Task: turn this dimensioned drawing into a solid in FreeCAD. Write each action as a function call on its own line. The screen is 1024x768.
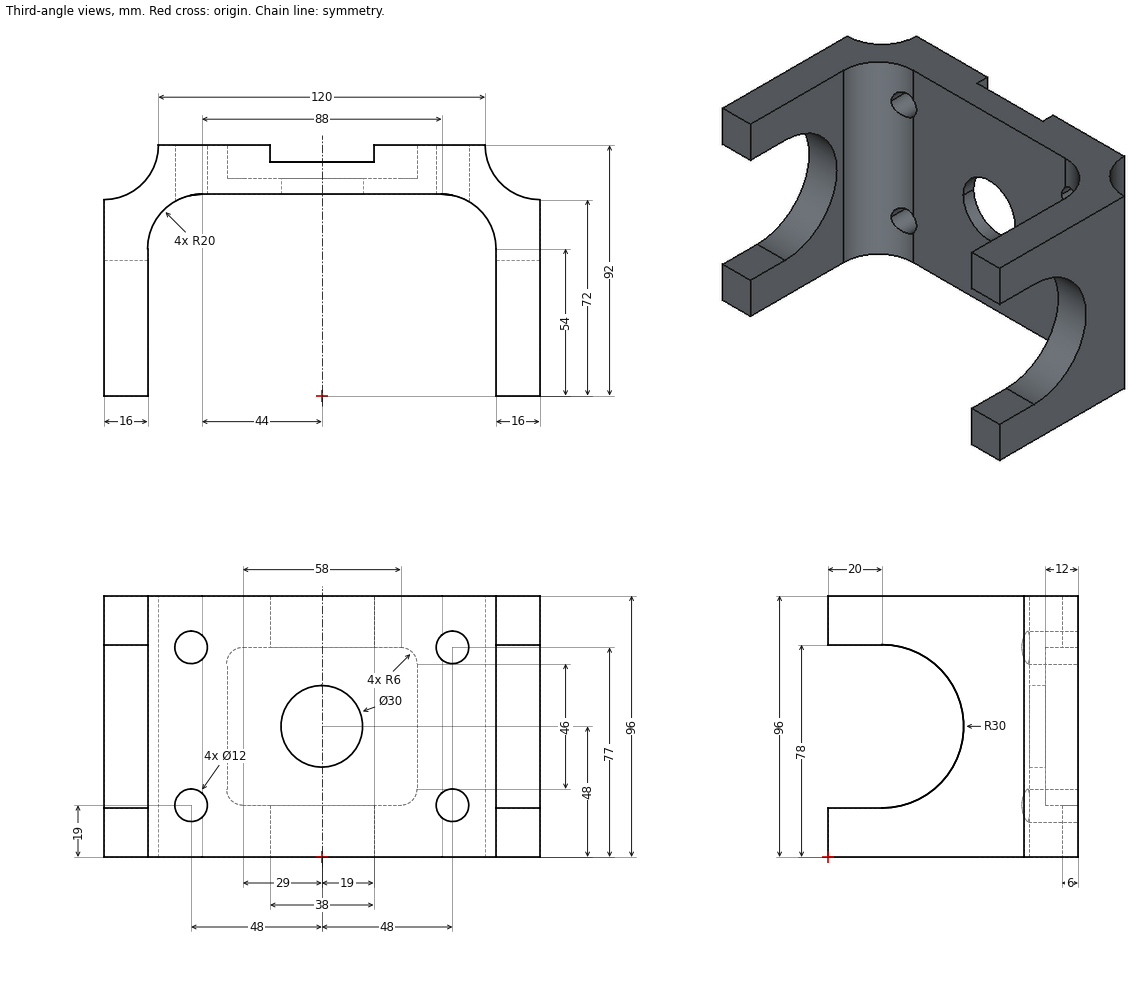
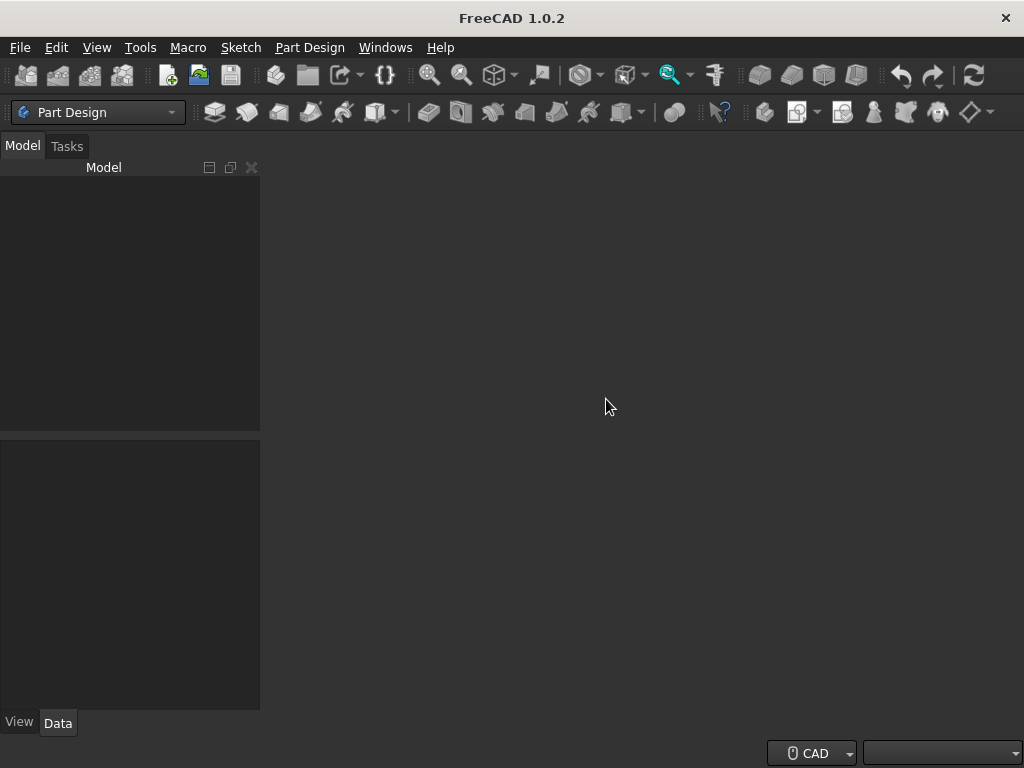
click(168, 76)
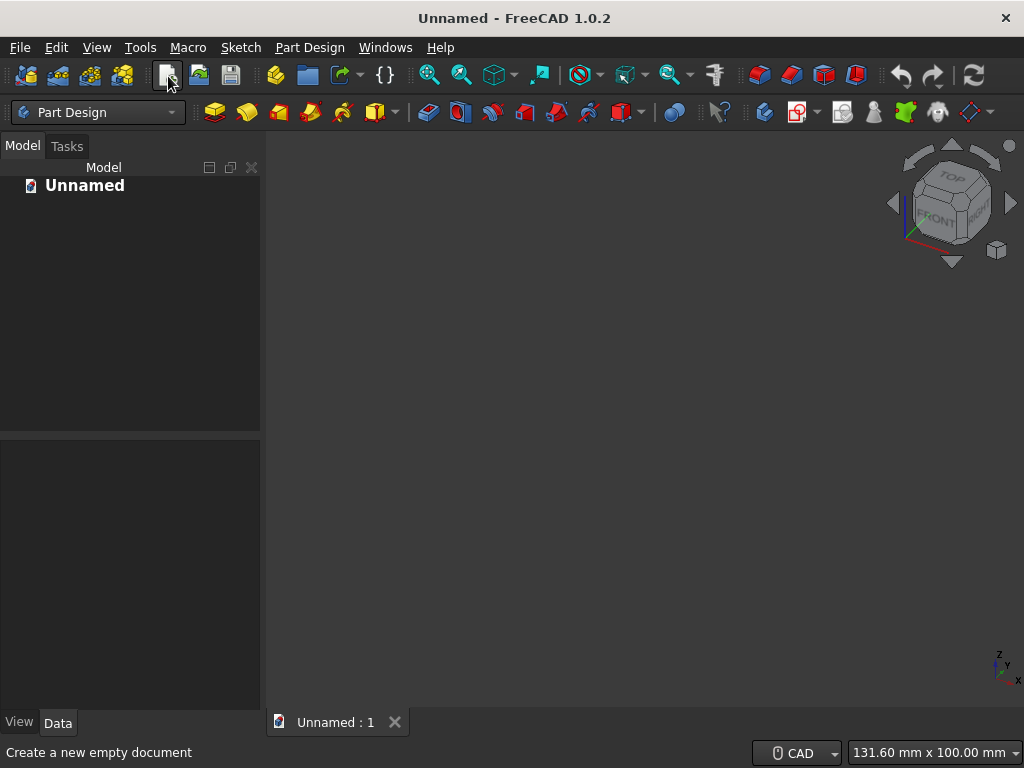
click(798, 112)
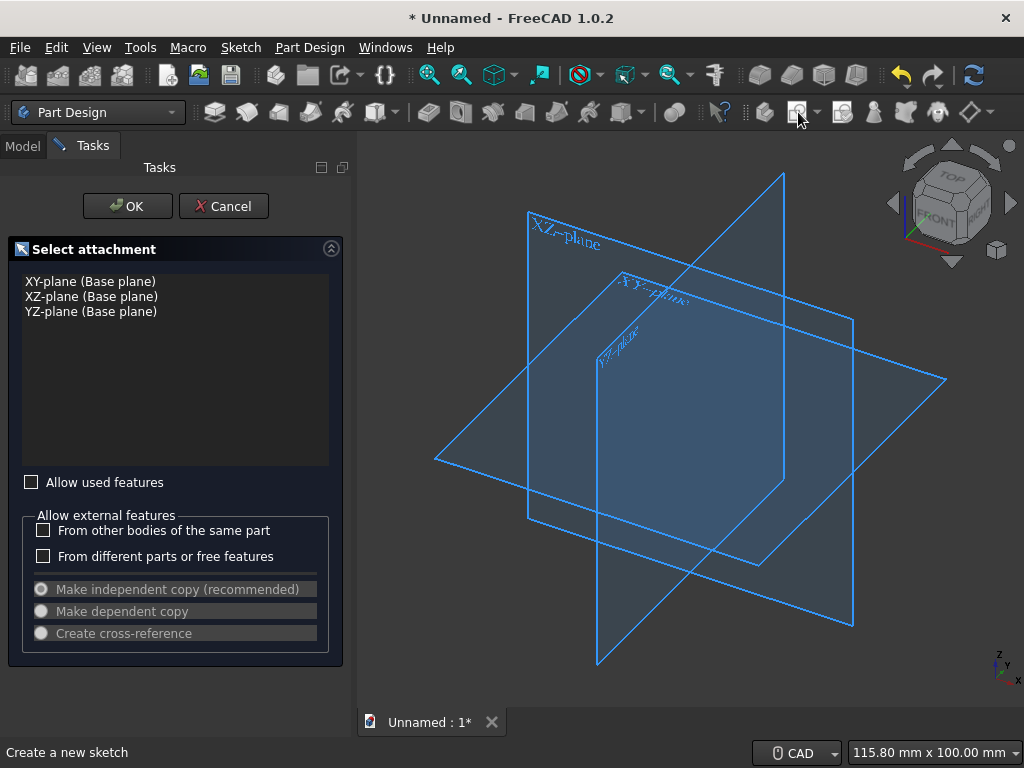
click(82, 282)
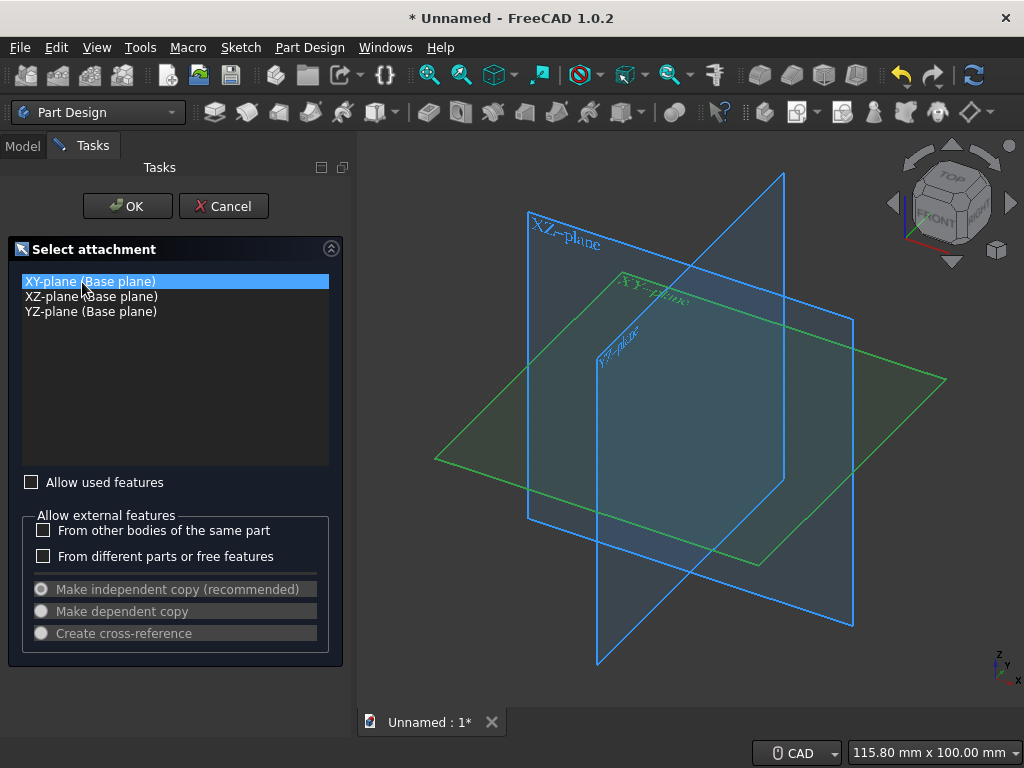
click(128, 206)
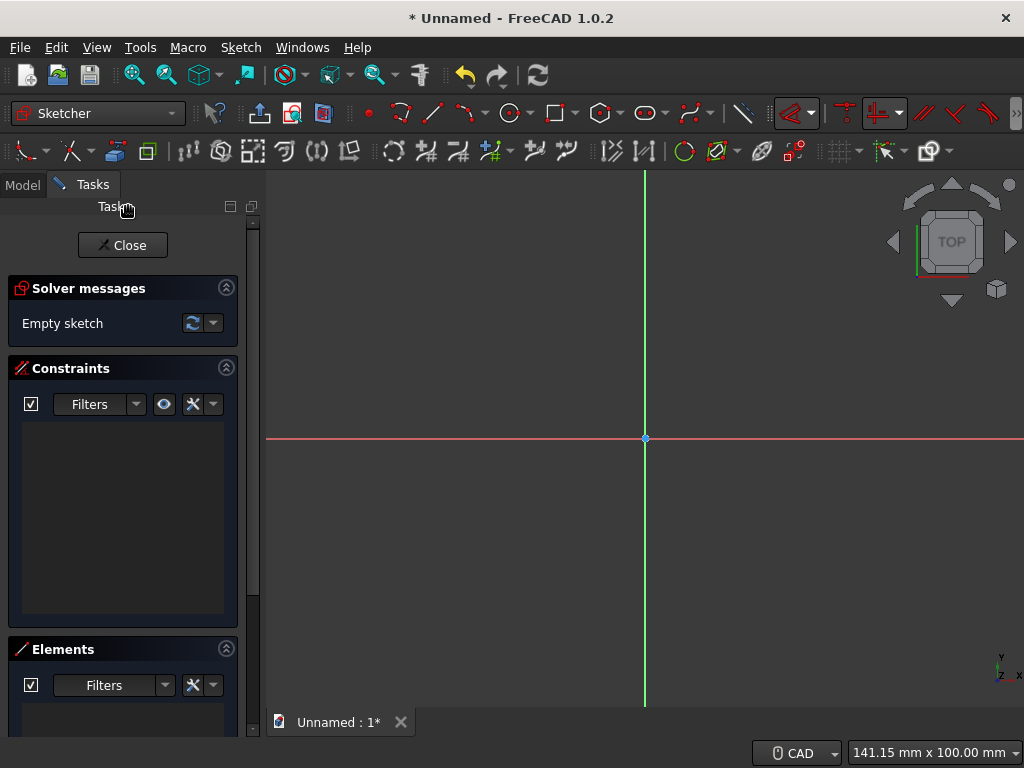
scroll(521, 640, down, 4)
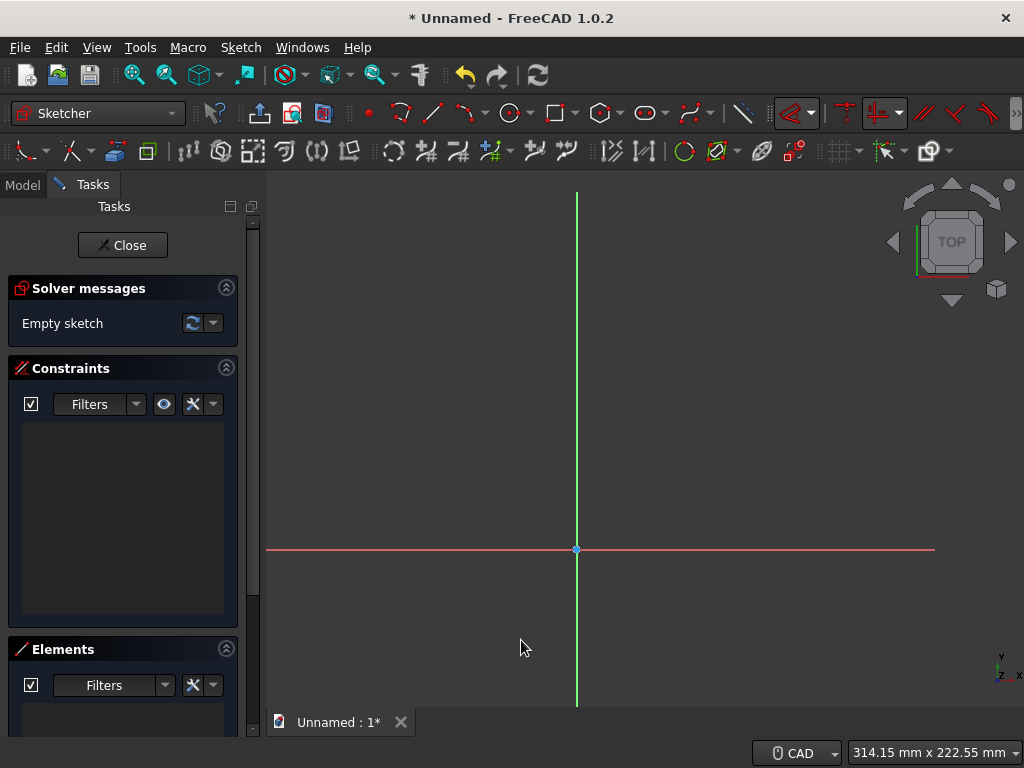
click(434, 114)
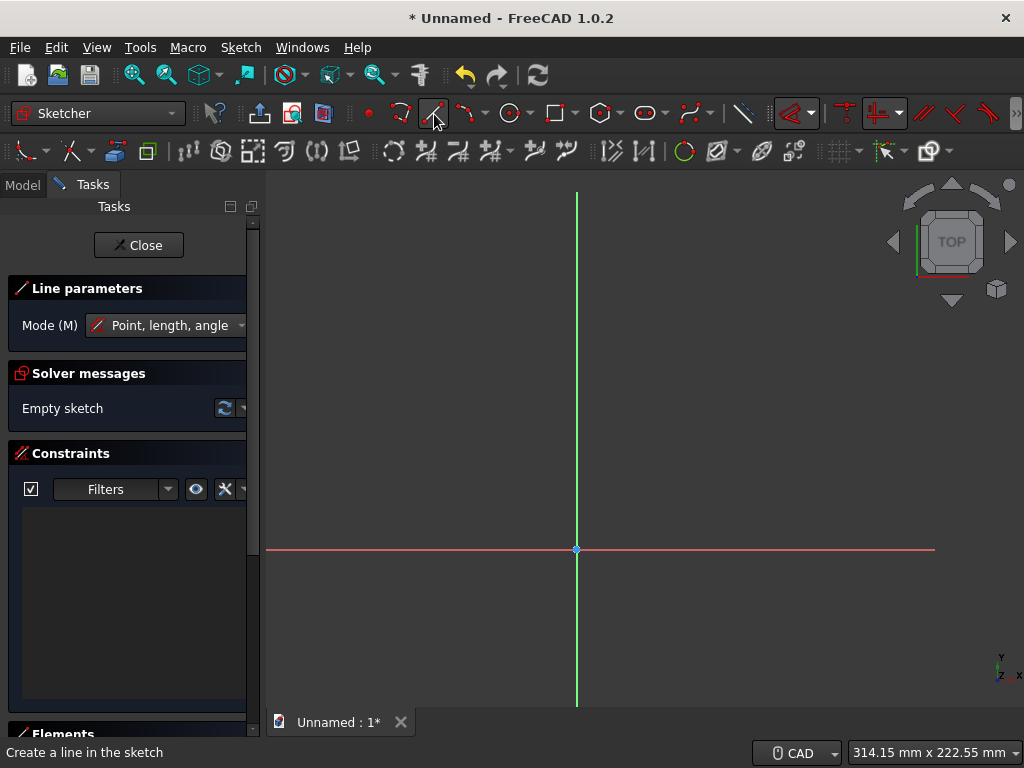
click(471, 371)
click(683, 371)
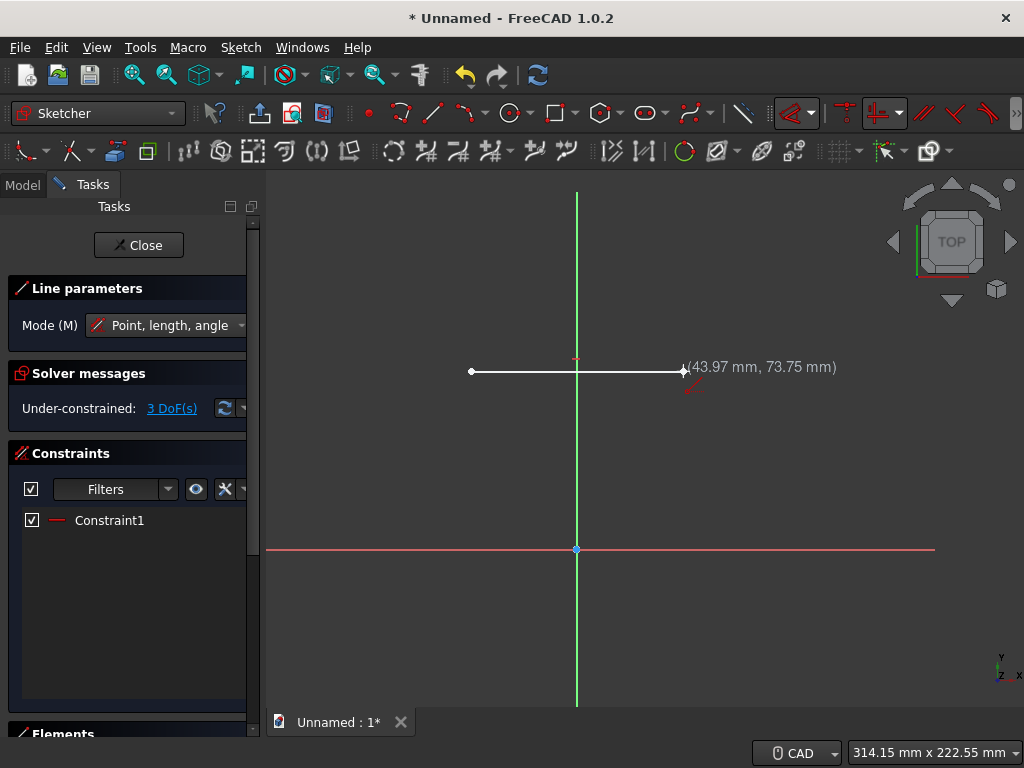
click(402, 114)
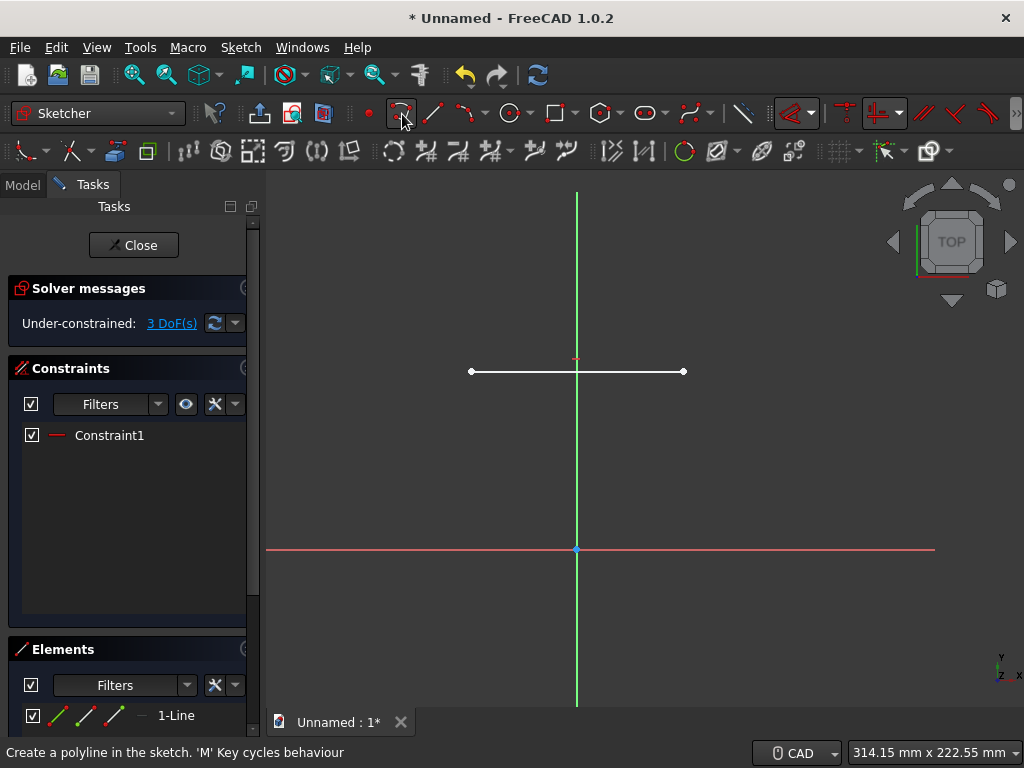
click(731, 420)
click(731, 550)
click(770, 541)
click(770, 376)
right_click(770, 376)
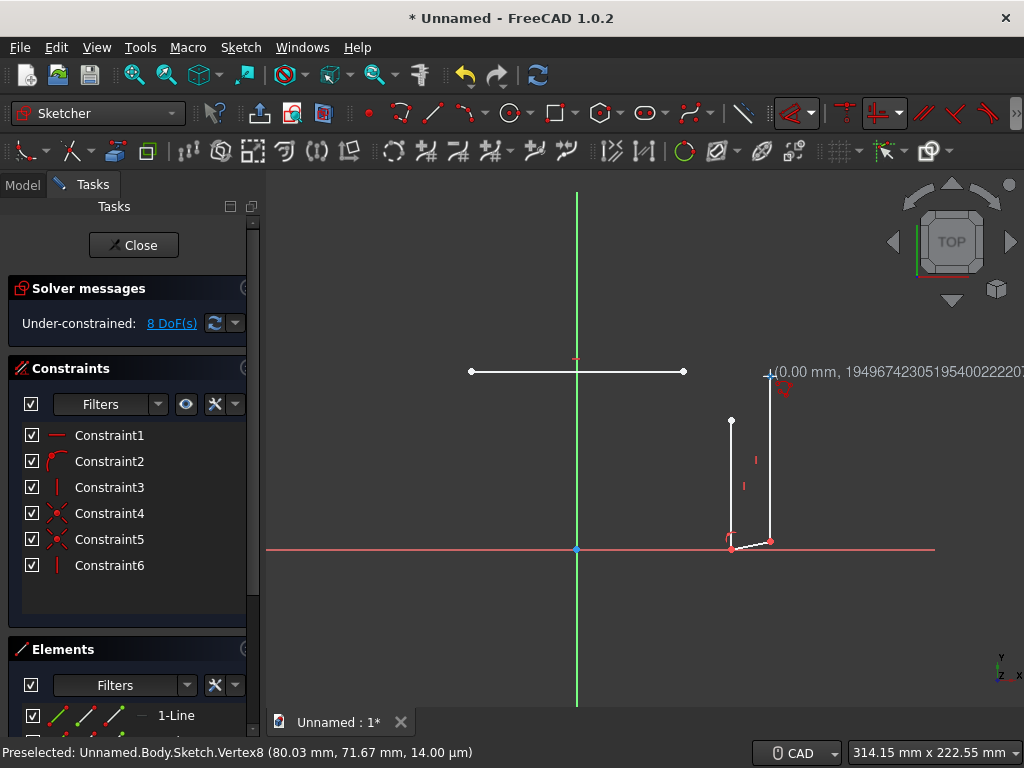
click(434, 114)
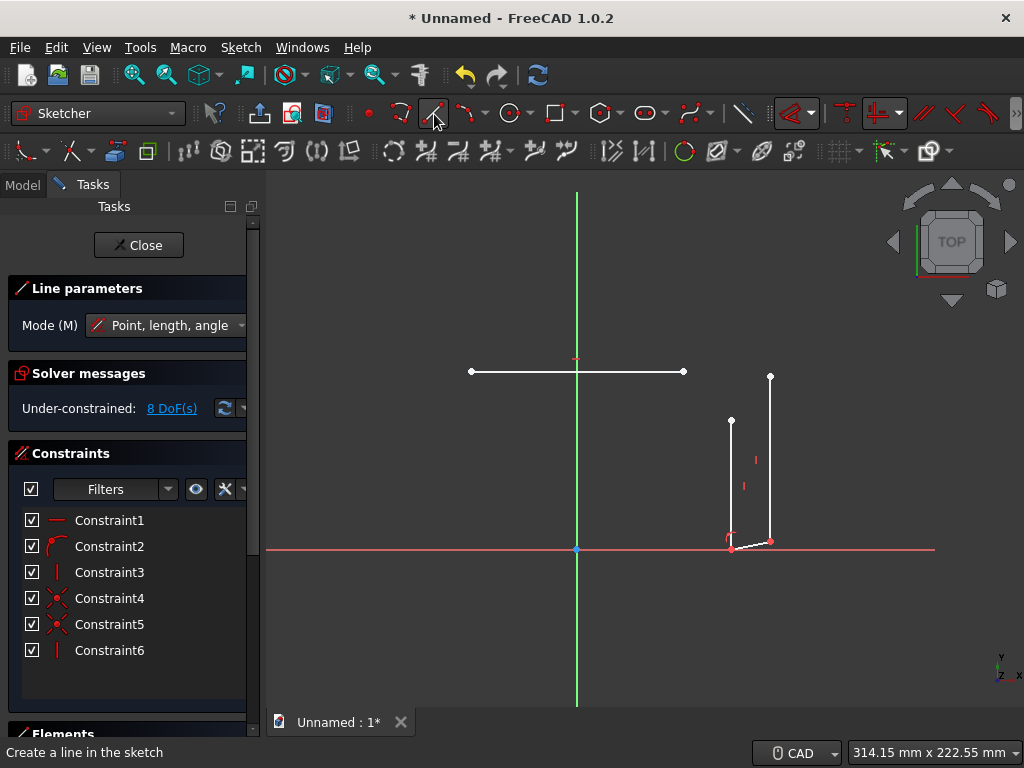
click(722, 328)
click(432, 328)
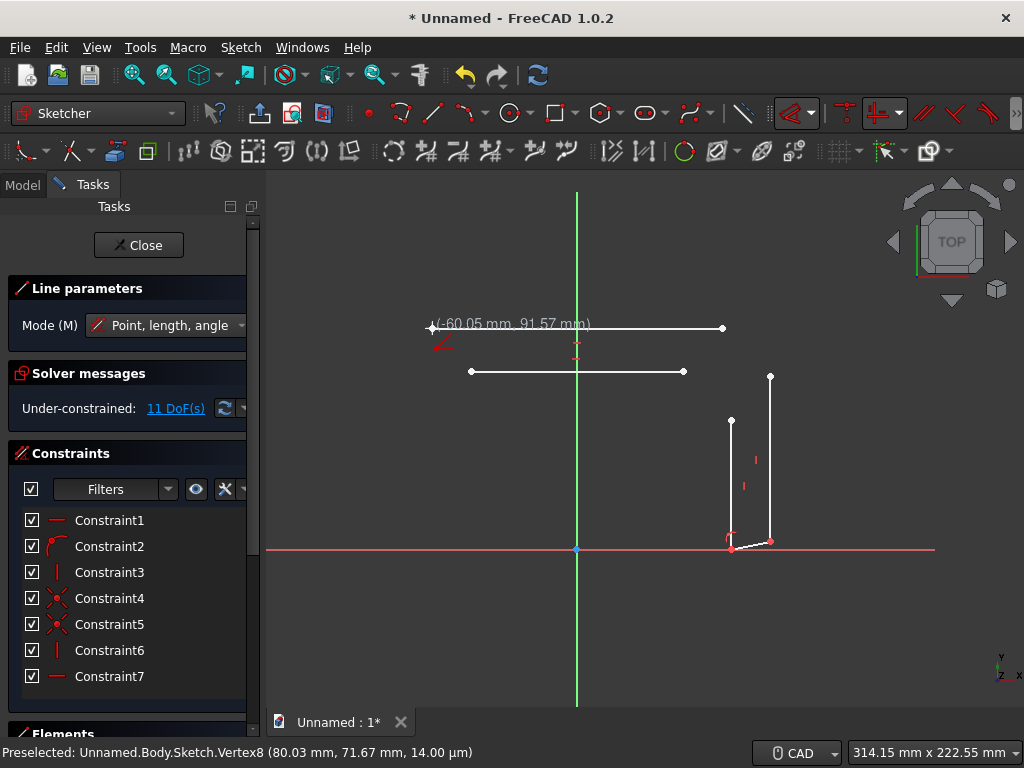
click(402, 114)